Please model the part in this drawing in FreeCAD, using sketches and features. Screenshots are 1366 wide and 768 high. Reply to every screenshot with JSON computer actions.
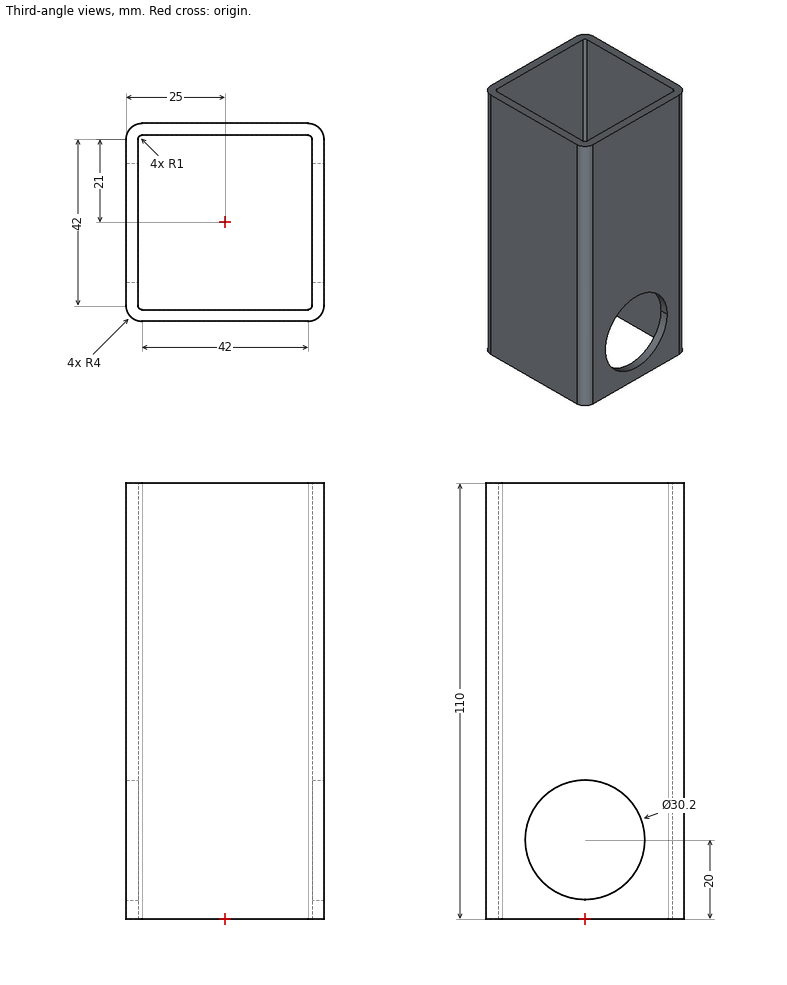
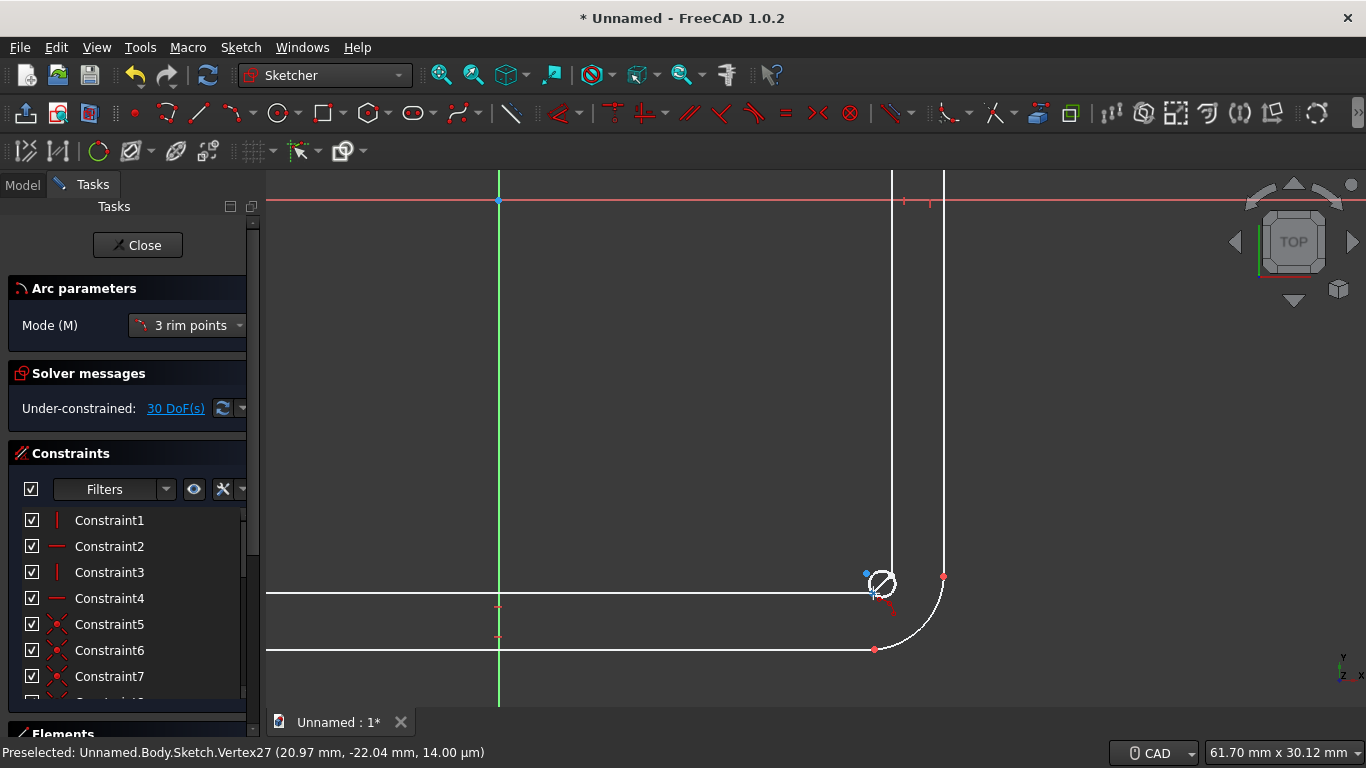
{"action": "scroll", "coordinate": [886, 587], "scroll_direction": "up", "scroll_amount": 6}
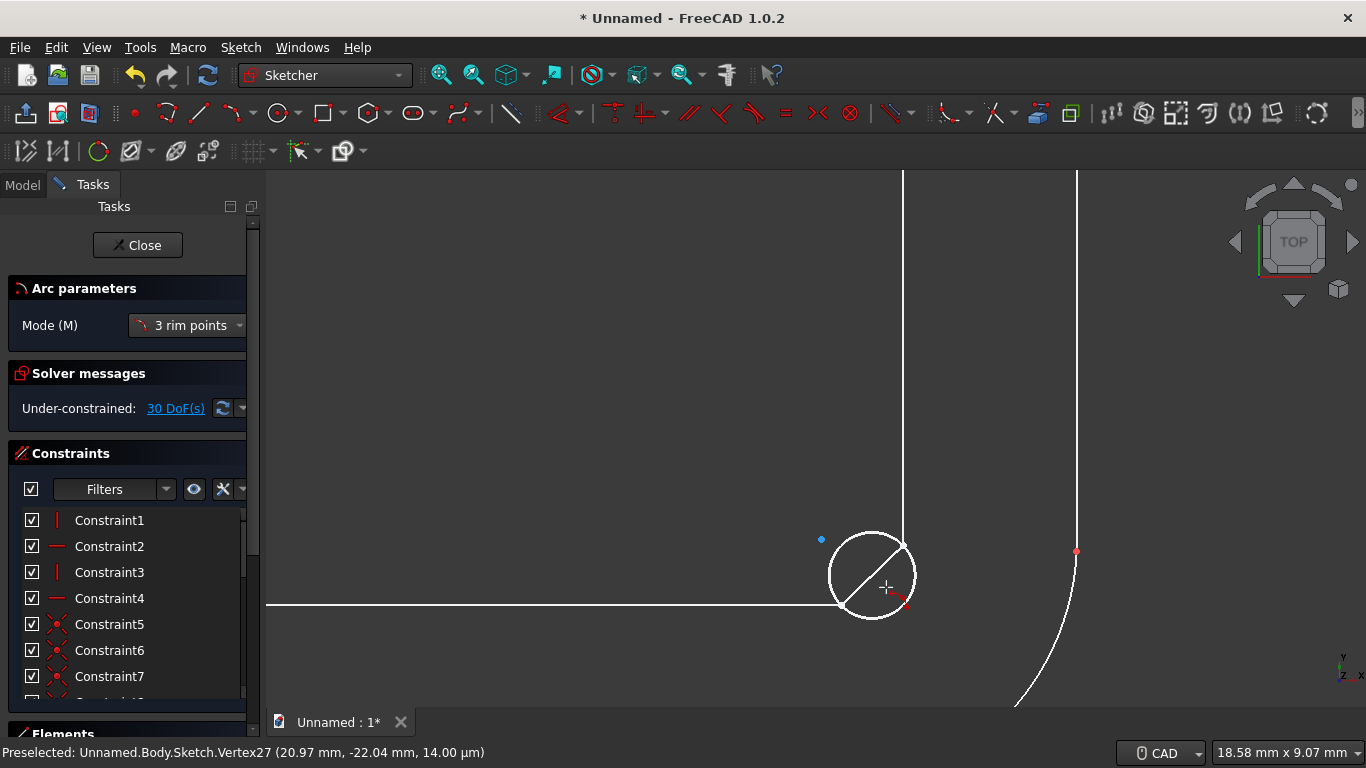
{"action": "left_click", "coordinate": [885, 585]}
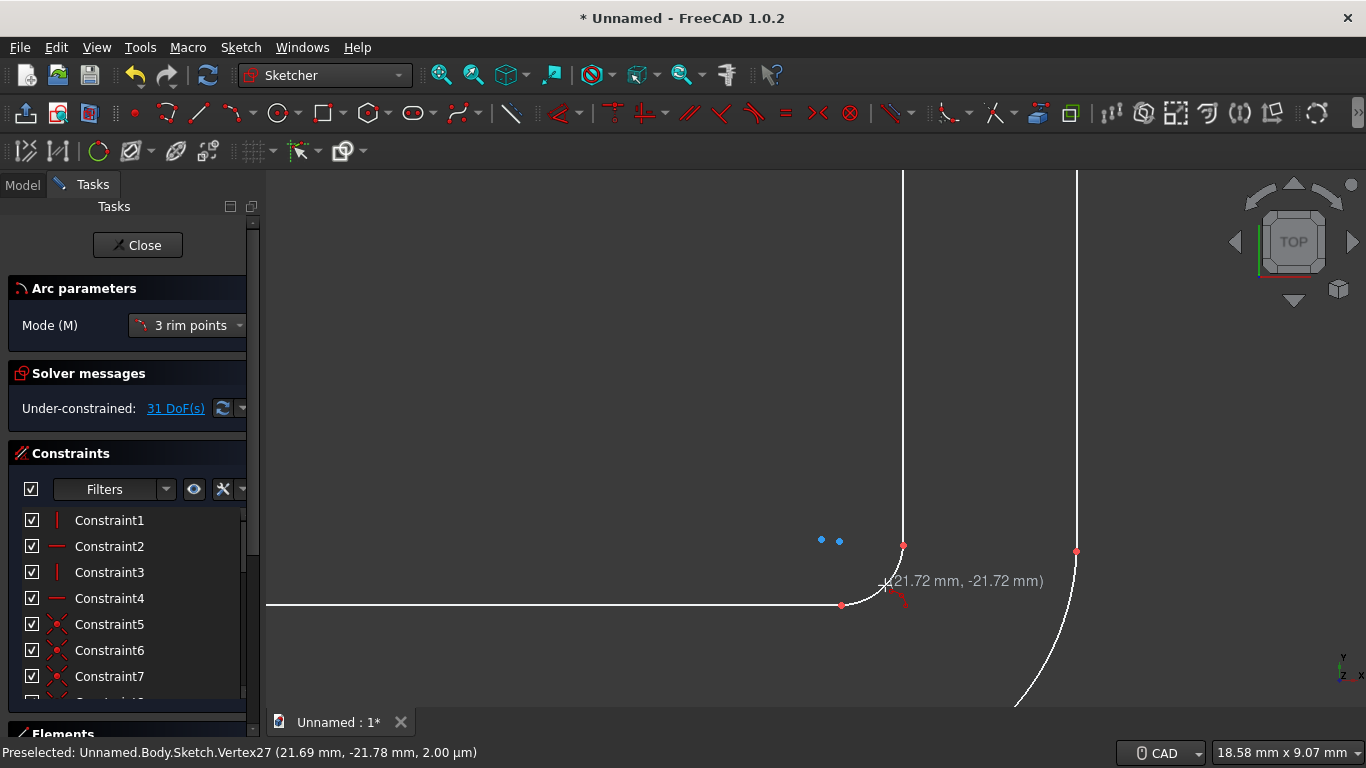
{"action": "scroll", "coordinate": [891, 580], "scroll_direction": "down", "scroll_amount": 11}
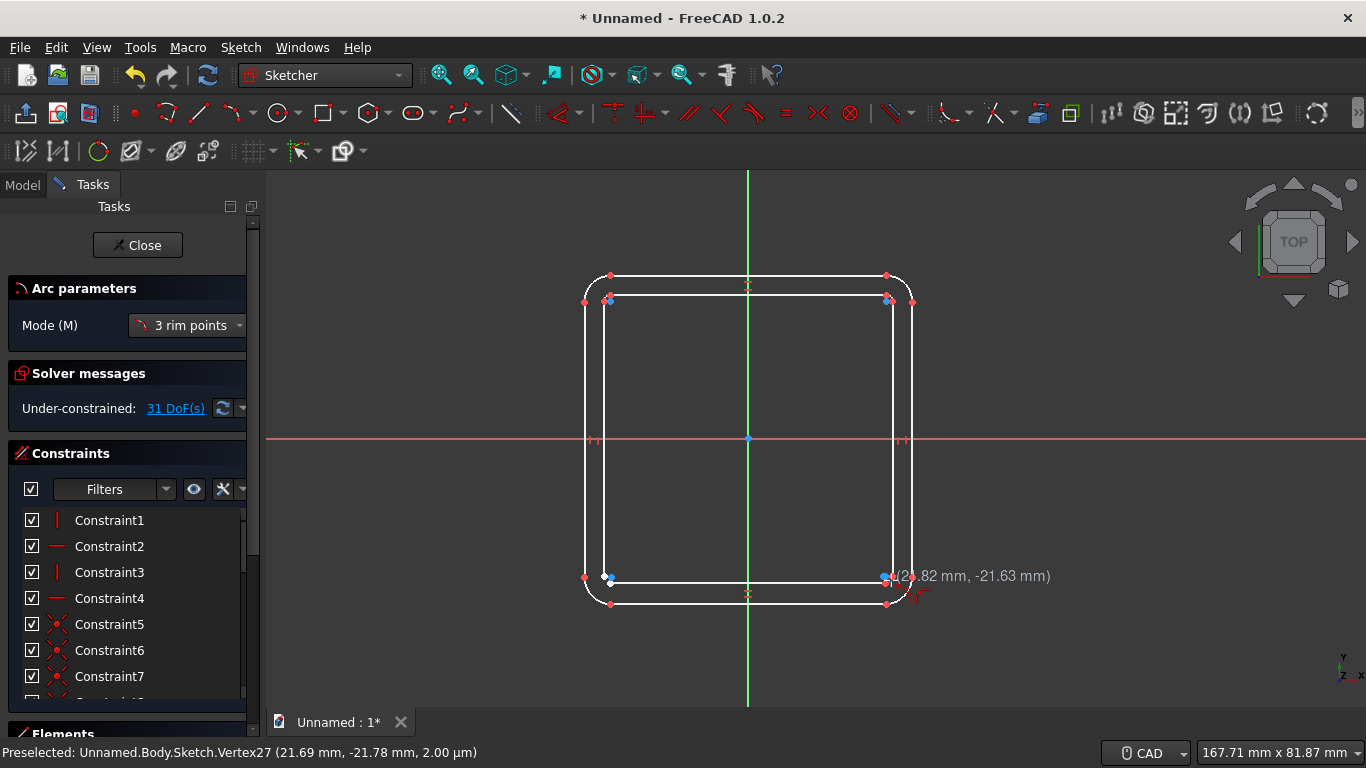
{"action": "scroll", "coordinate": [611, 583], "scroll_direction": "up", "scroll_amount": 5}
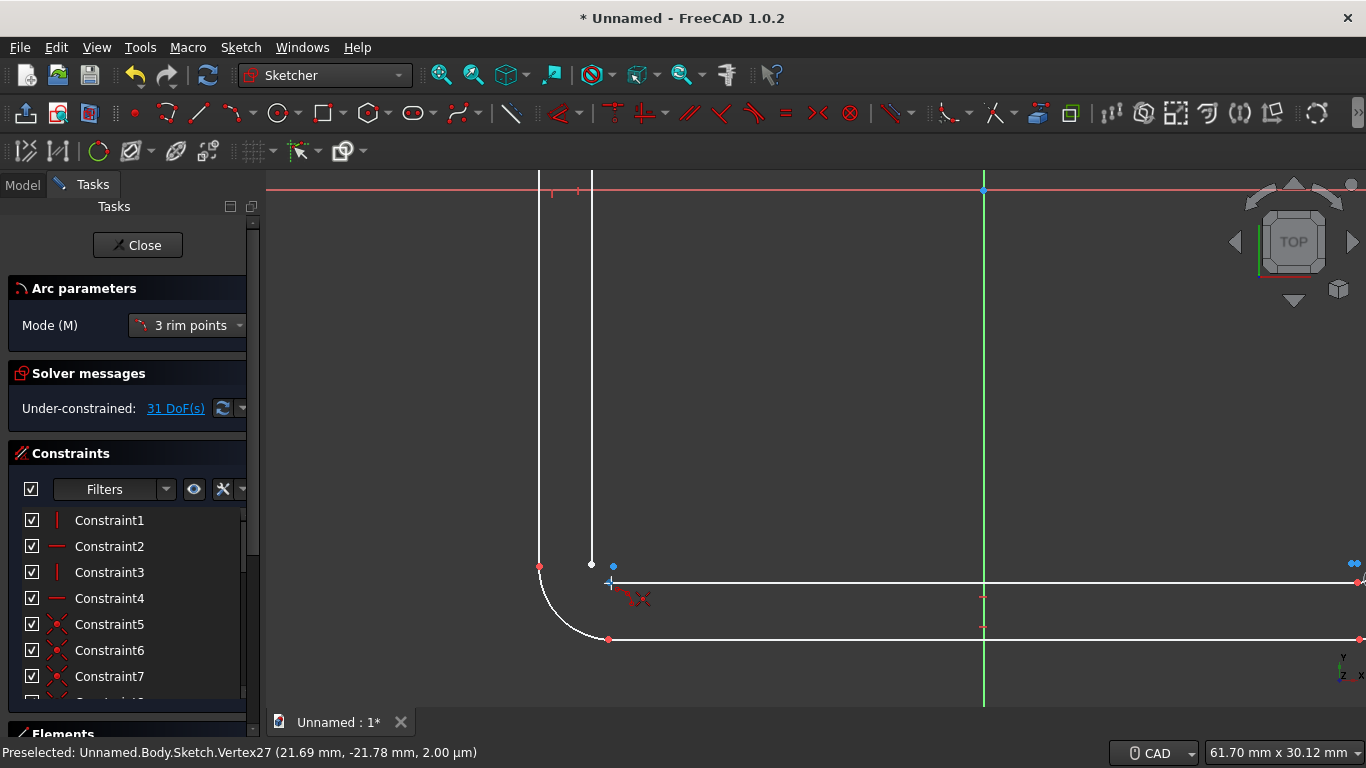
{"action": "left_click", "coordinate": [610, 583]}
{"action": "left_click", "coordinate": [592, 565]}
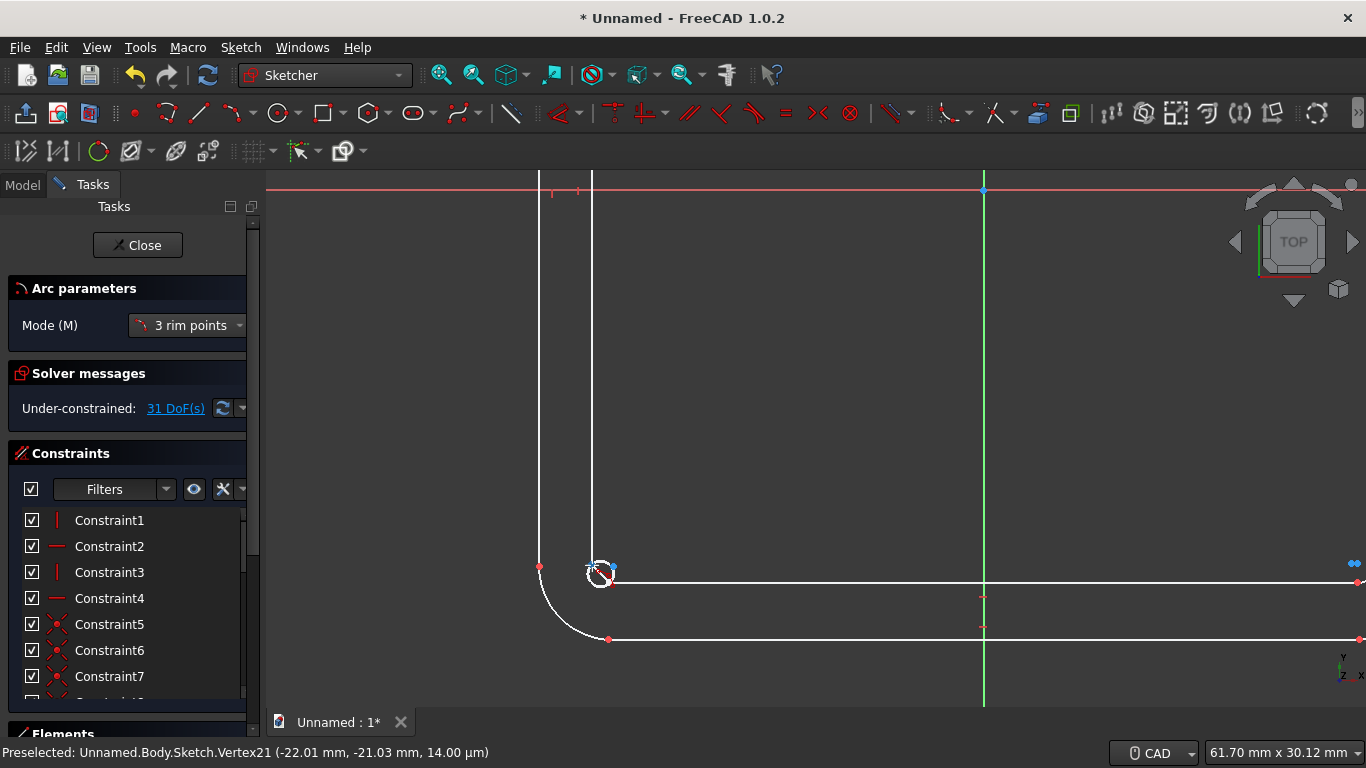
{"action": "scroll", "coordinate": [597, 577], "scroll_direction": "up", "scroll_amount": 6}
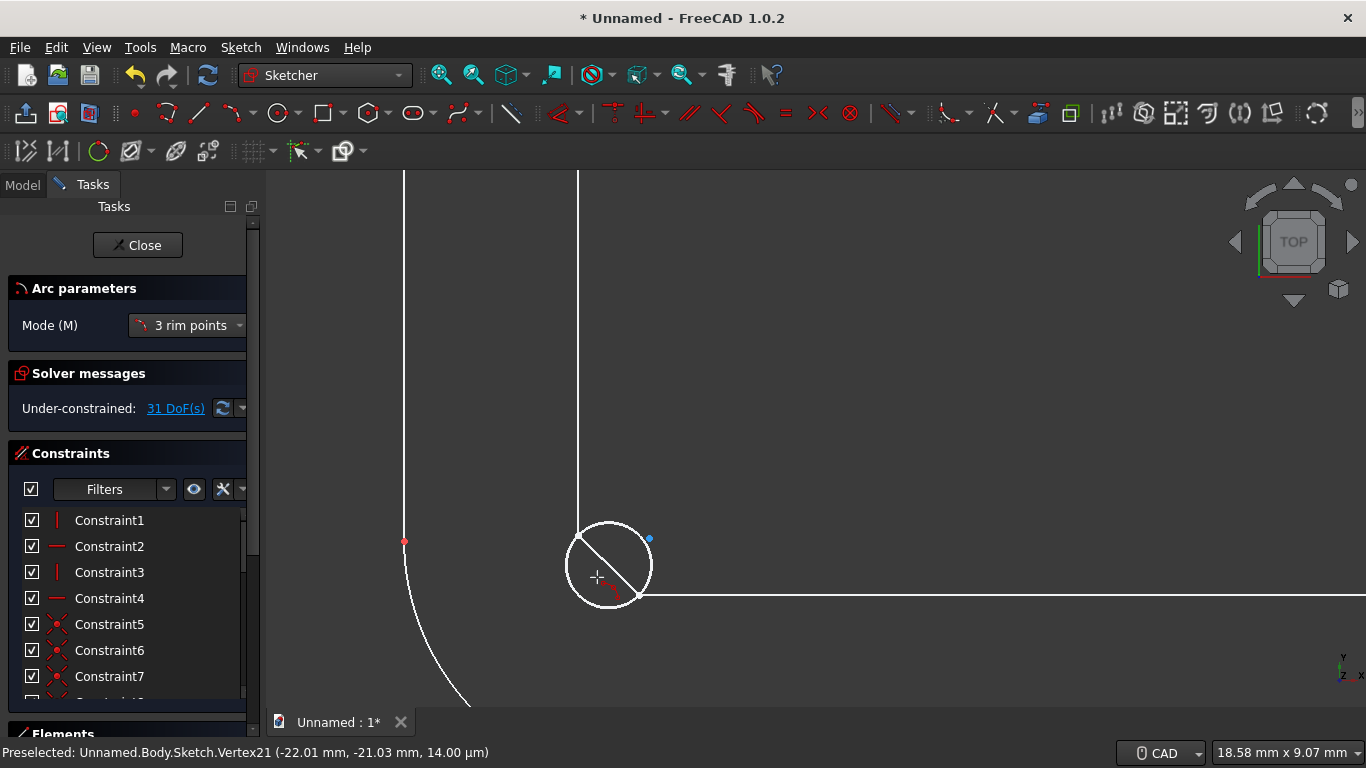
{"action": "left_click", "coordinate": [596, 575]}
{"action": "key", "text": "Escape"}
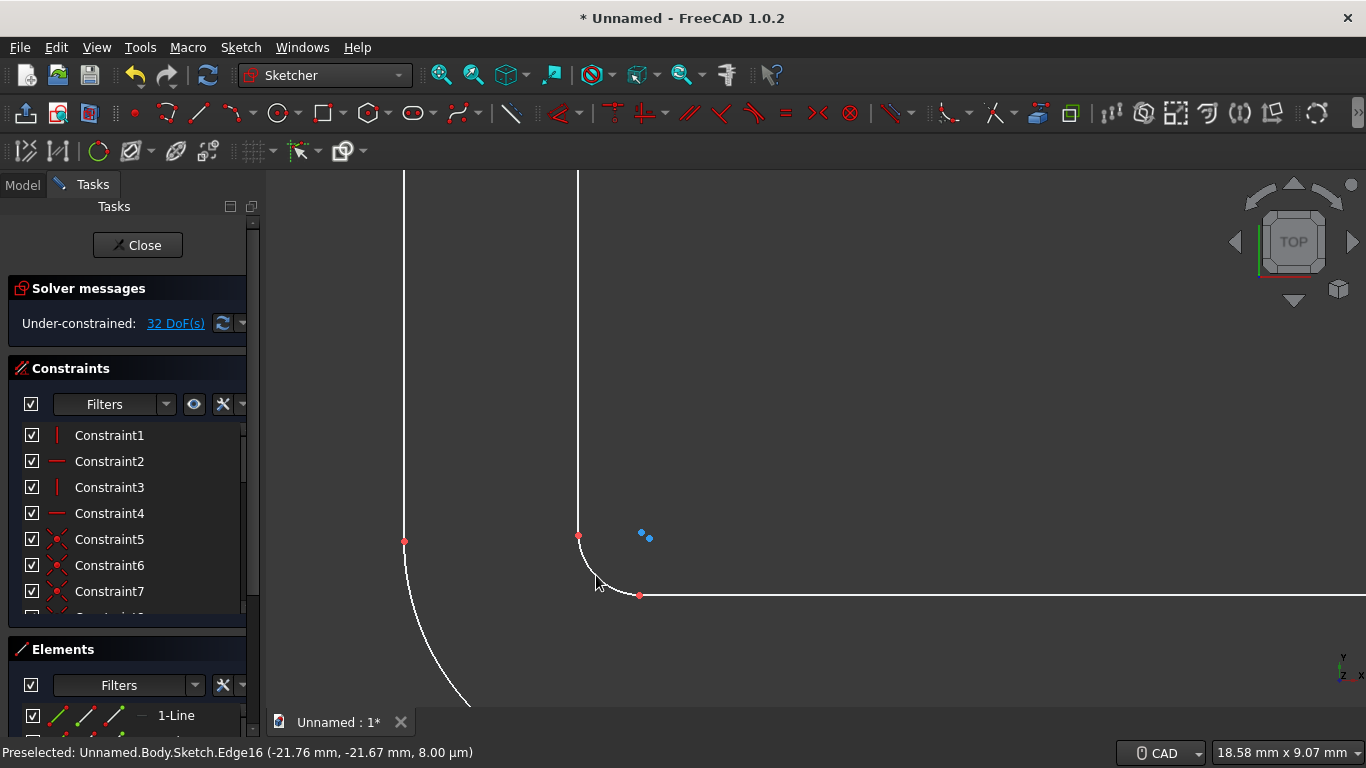
{"action": "scroll", "coordinate": [606, 582], "scroll_direction": "down", "scroll_amount": 11}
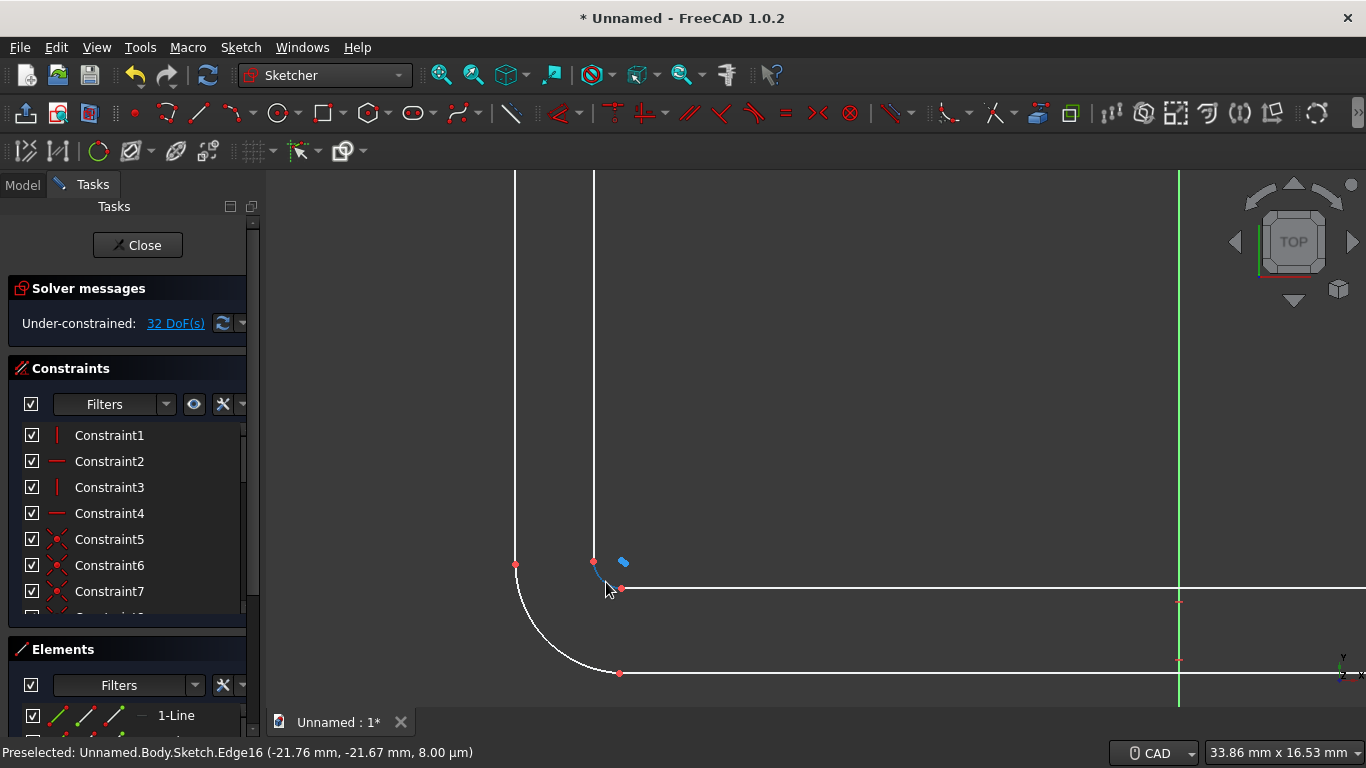
{"action": "left_click", "coordinate": [584, 386]}